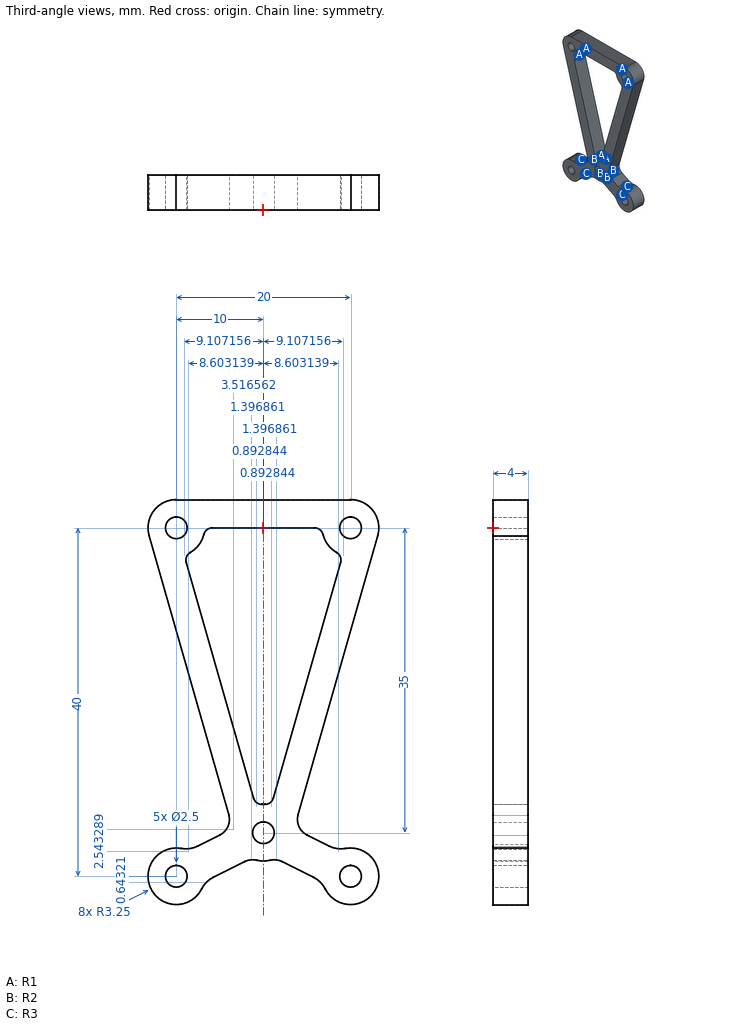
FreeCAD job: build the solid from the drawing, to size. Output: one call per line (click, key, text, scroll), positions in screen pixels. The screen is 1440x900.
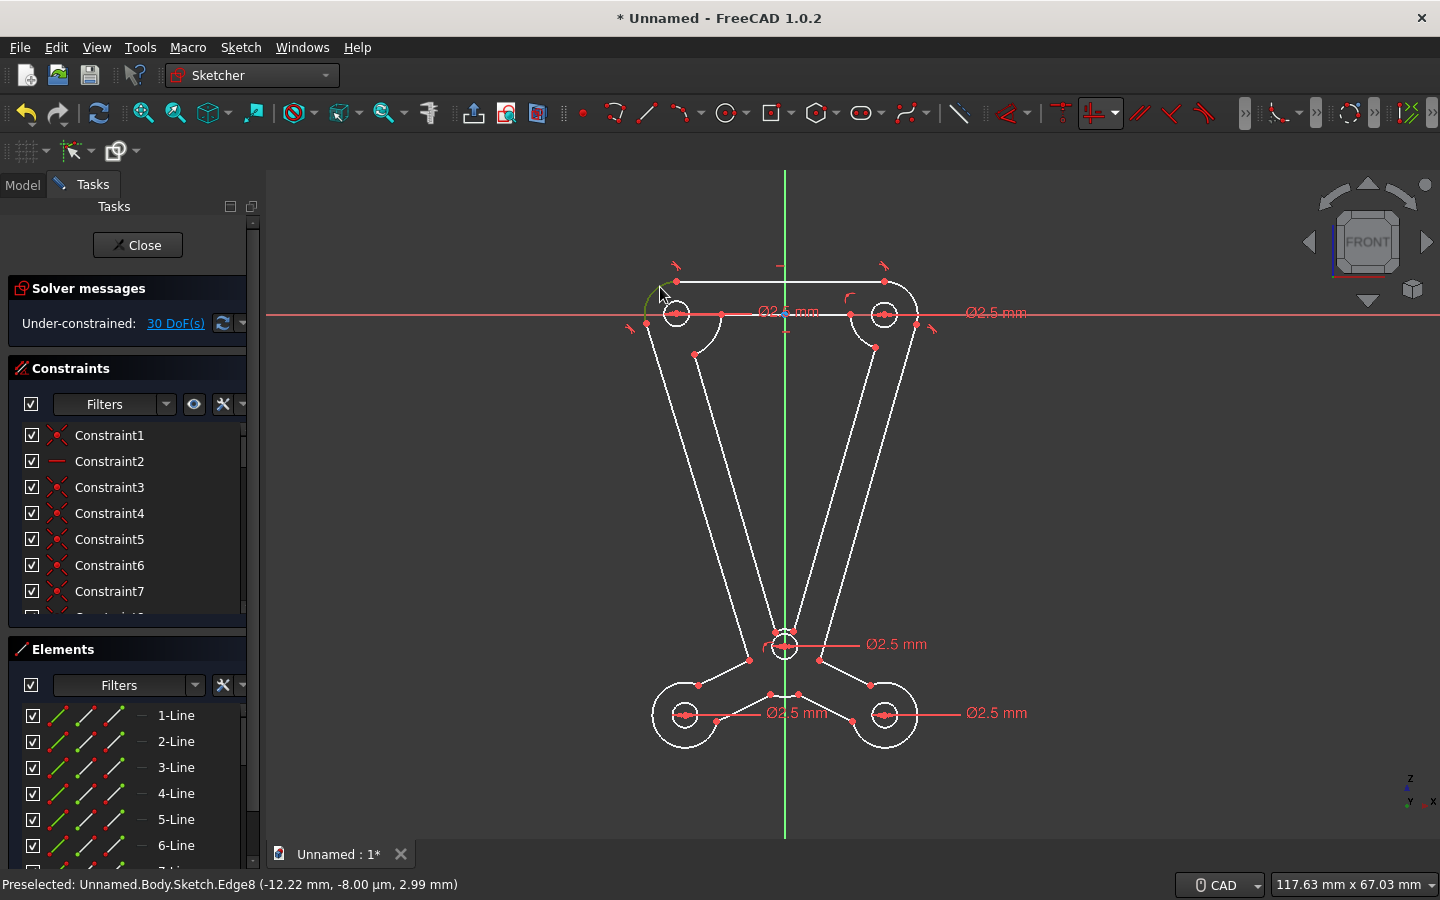
click(902, 287)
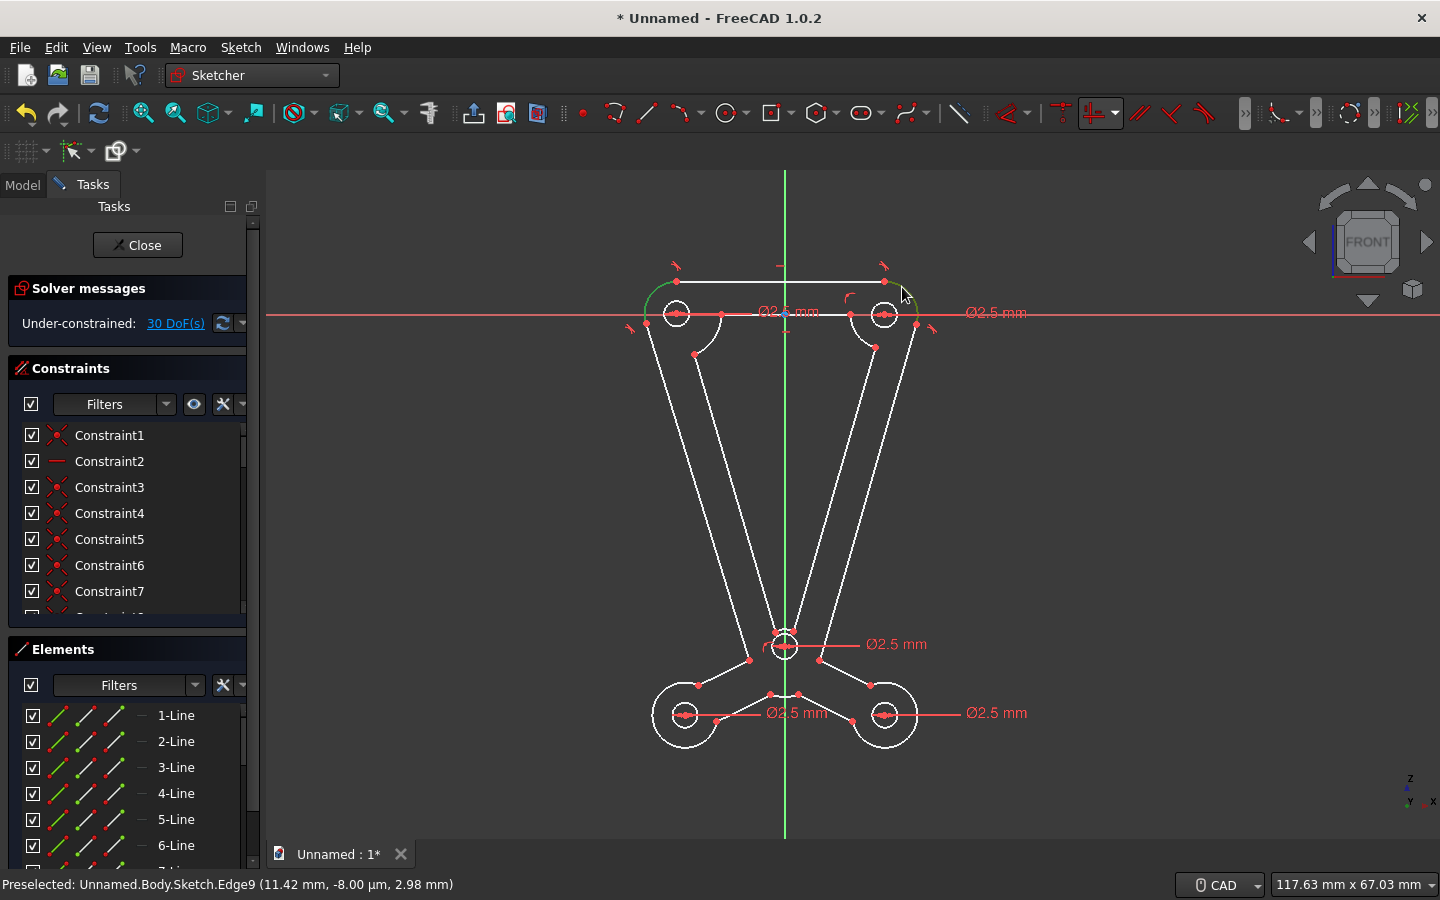
click(889, 748)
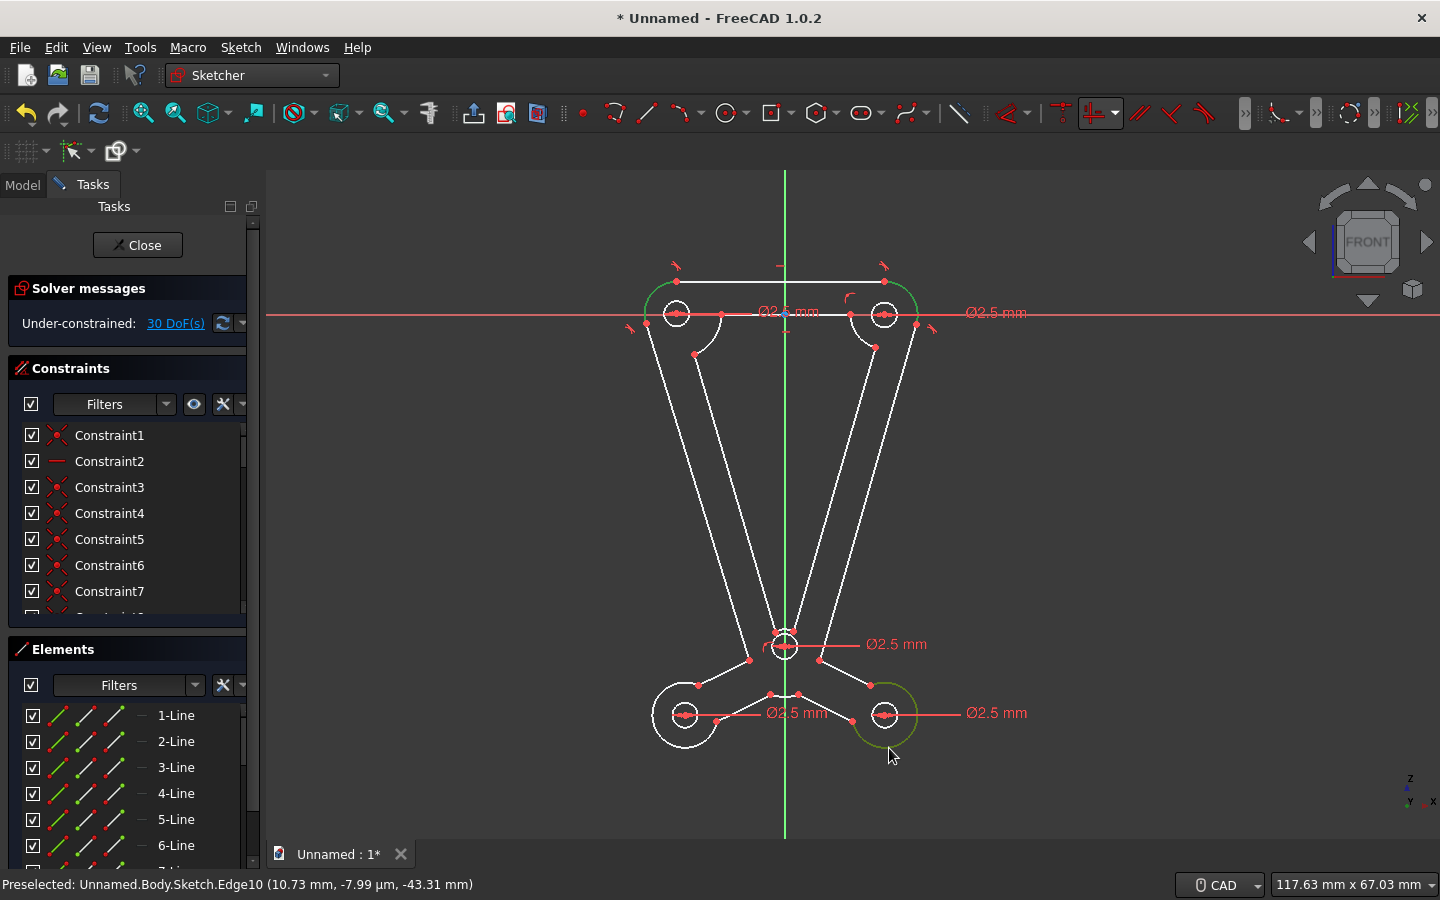
click(785, 697)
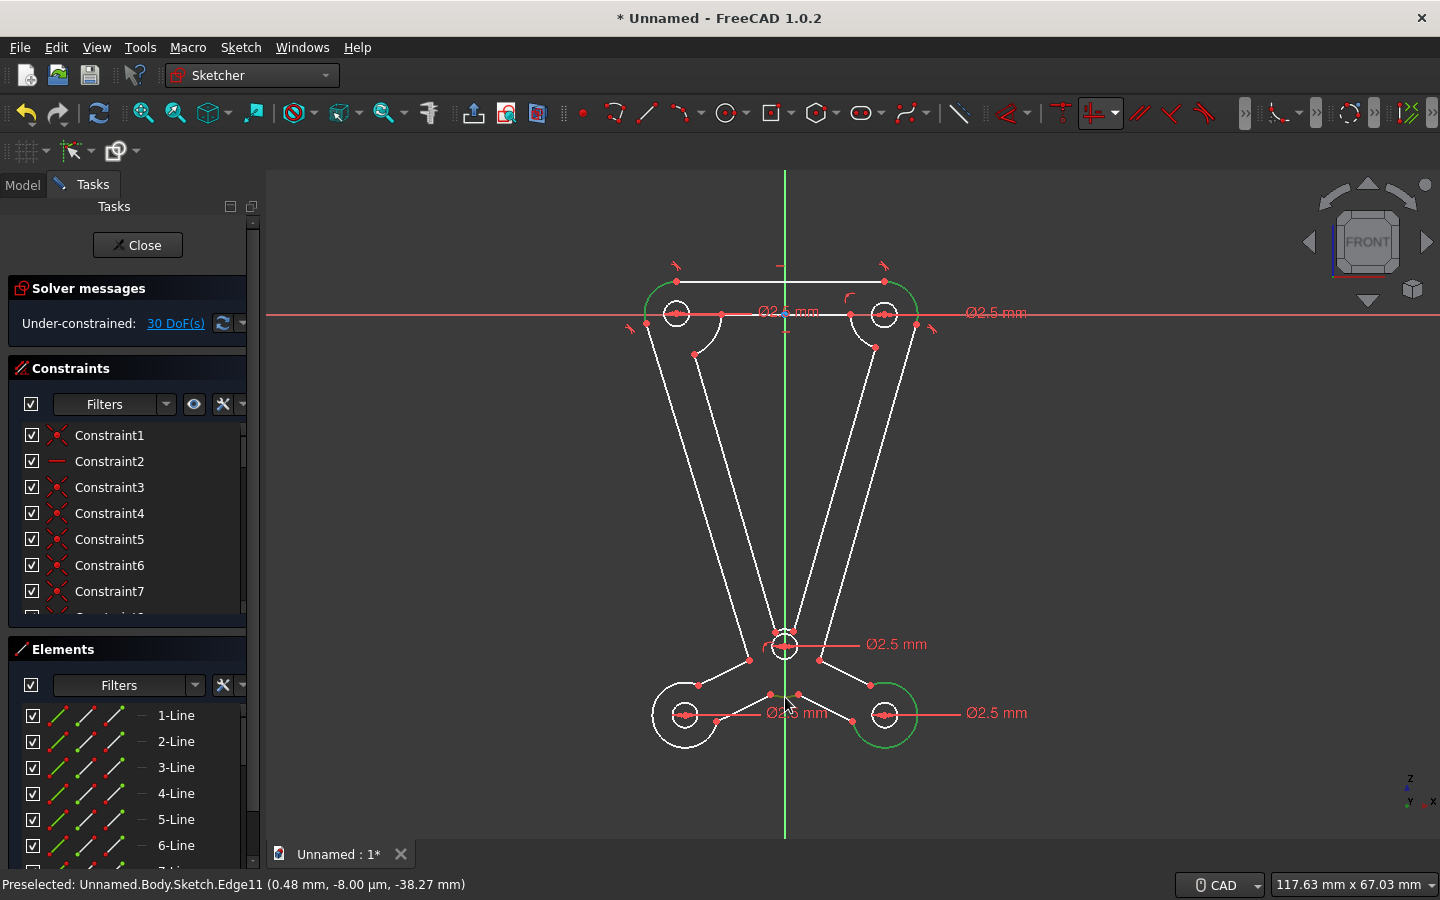
click(657, 699)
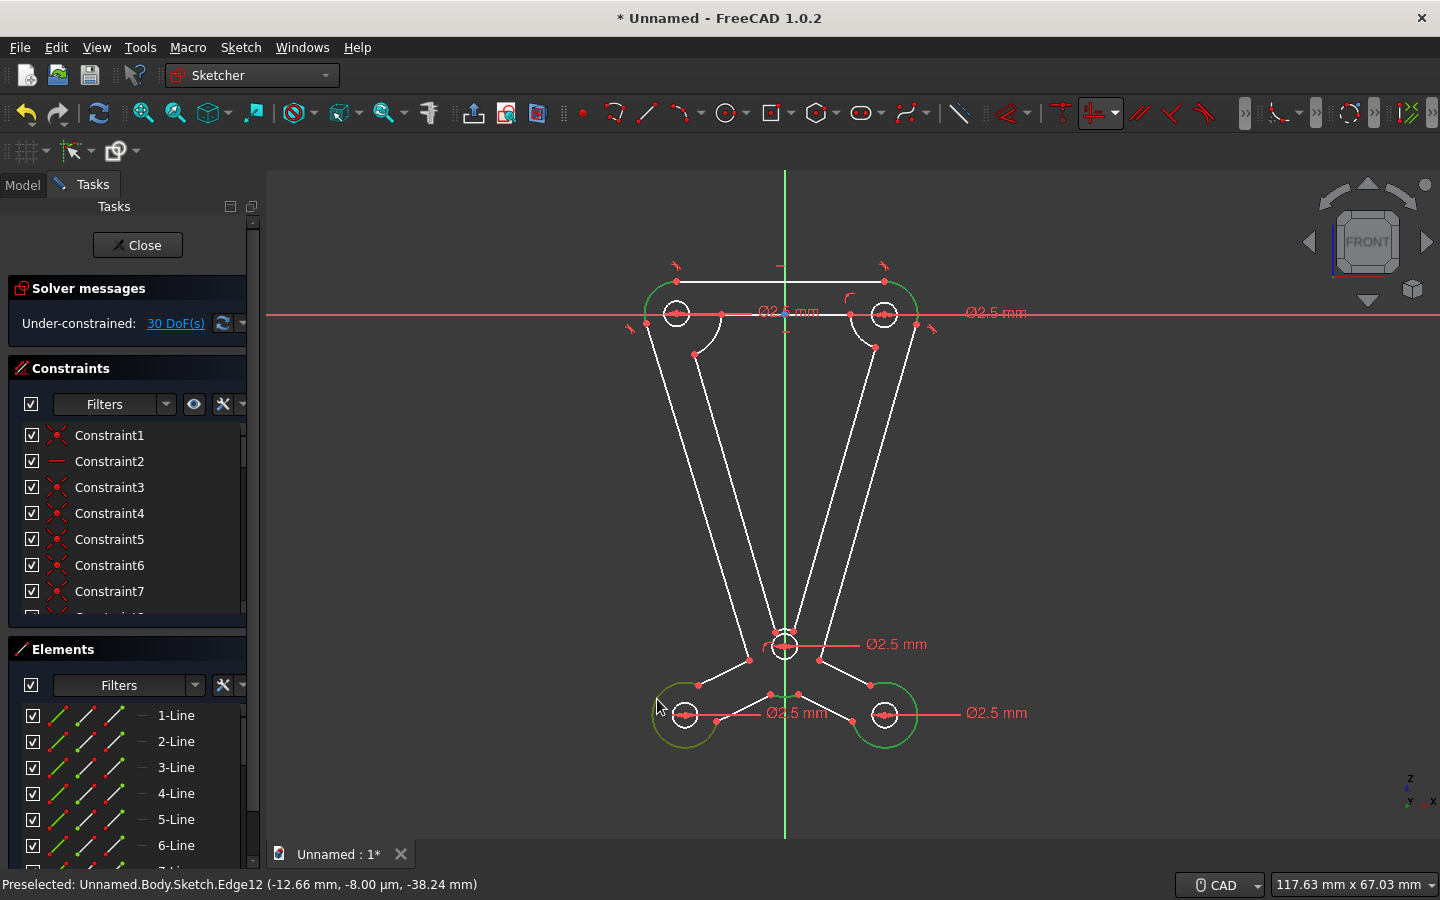
click(853, 328)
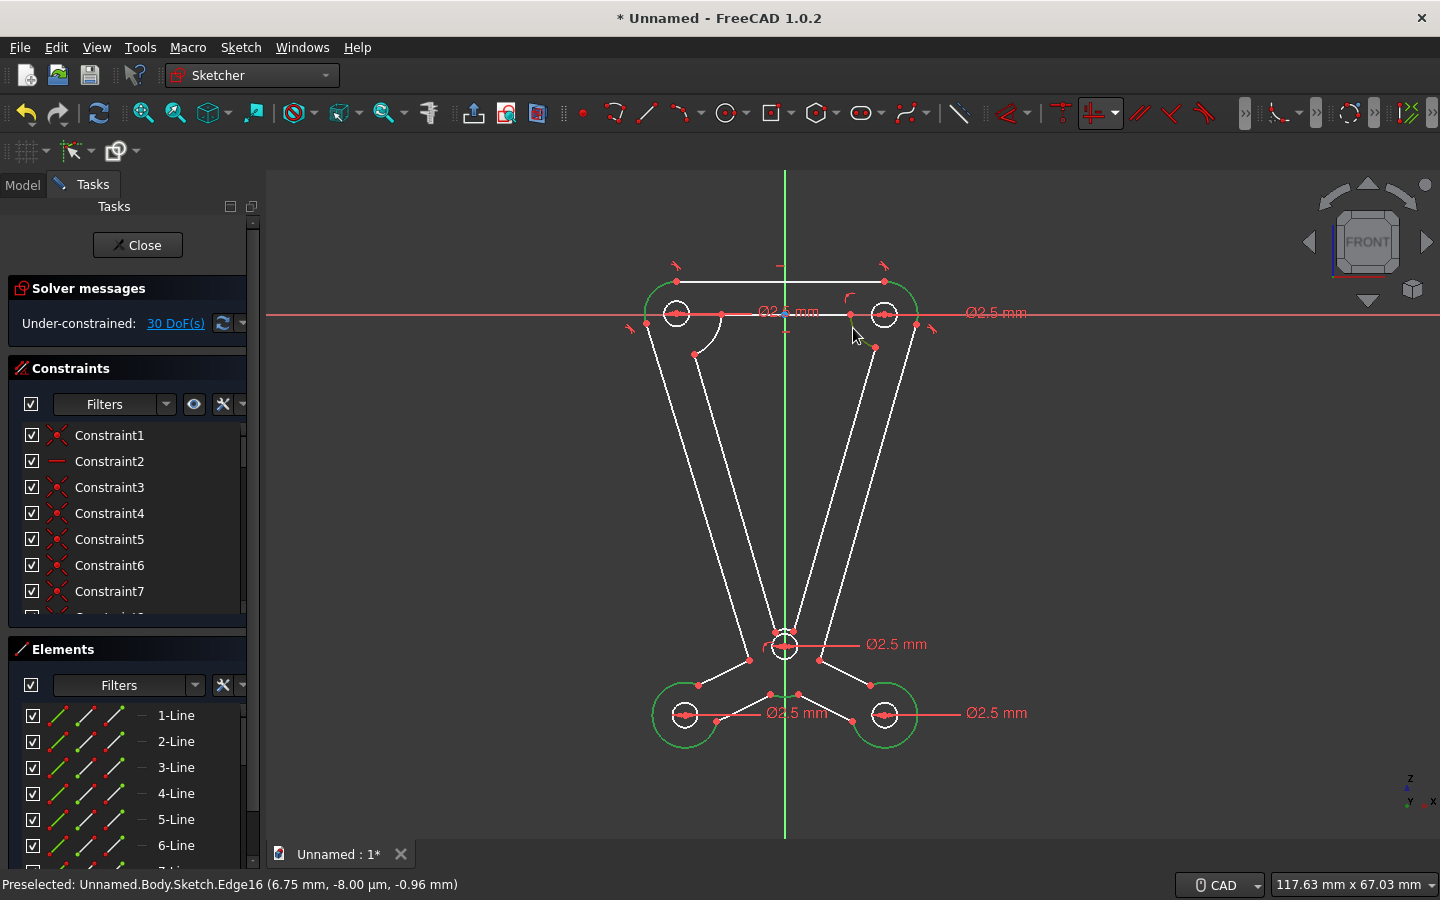
click(707, 346)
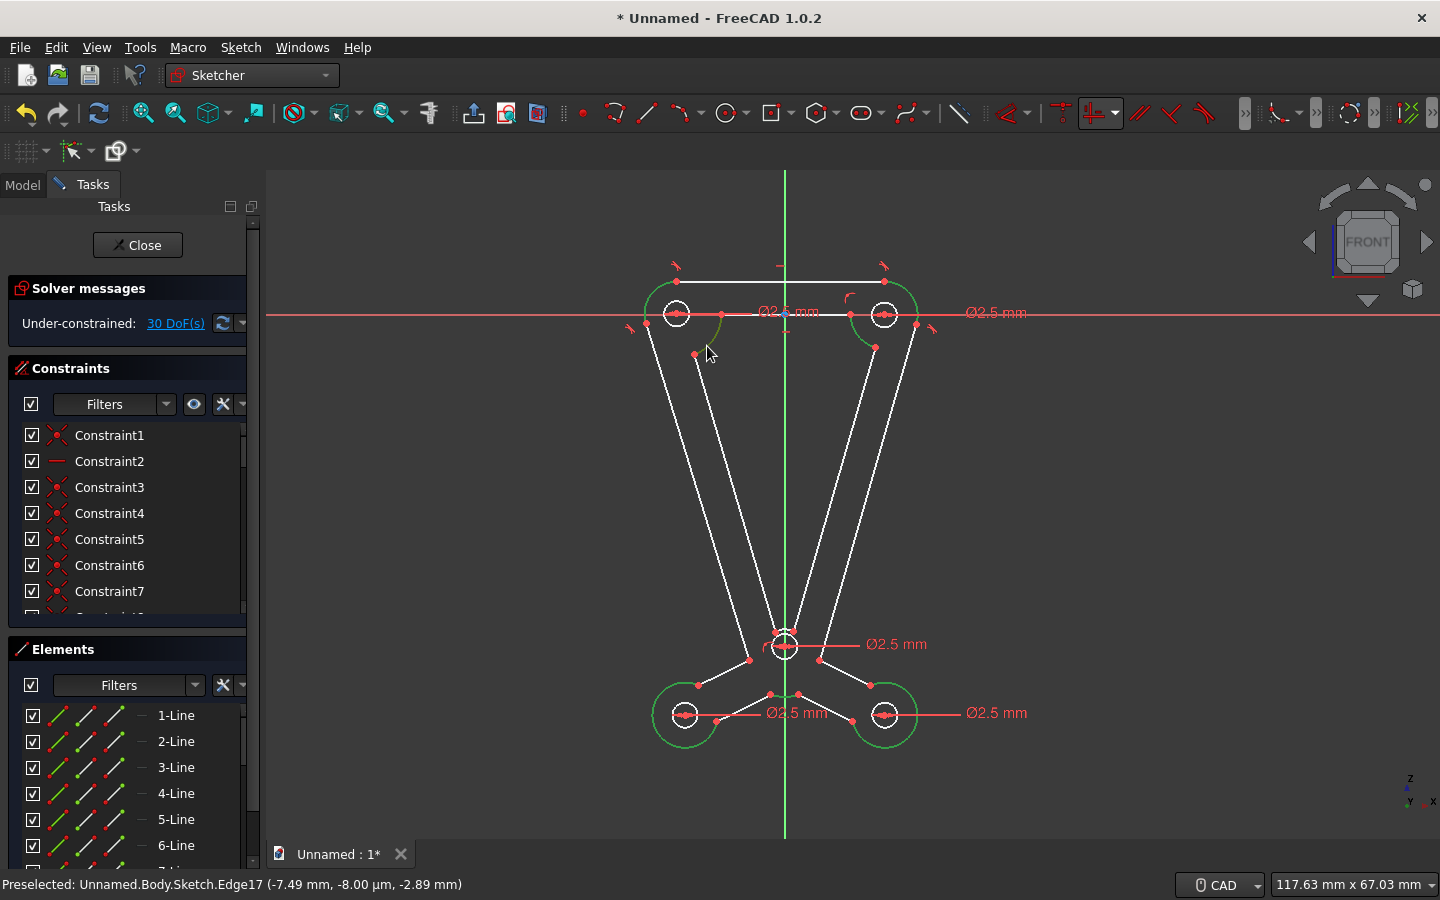
scroll(785, 629, up, 6)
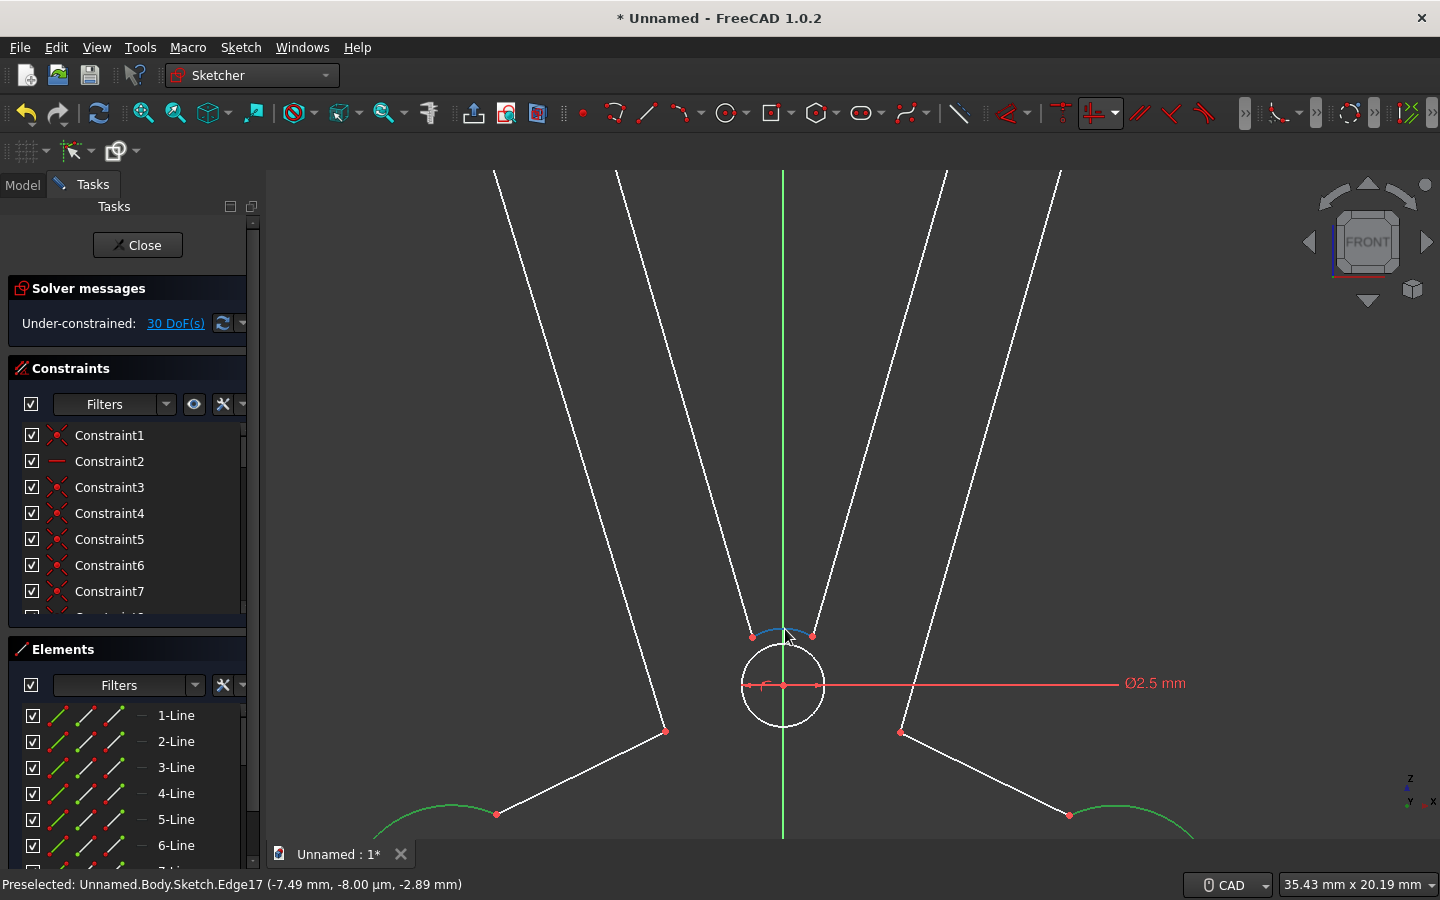
click(783, 629)